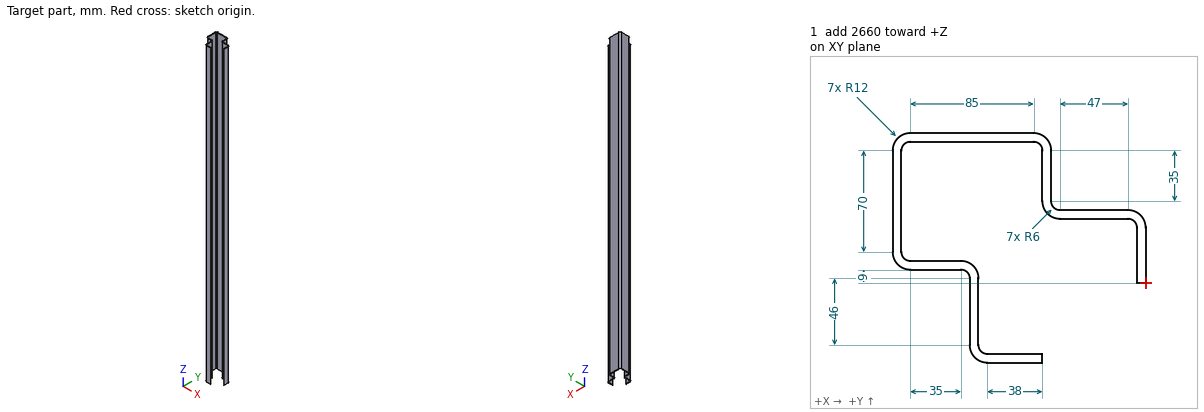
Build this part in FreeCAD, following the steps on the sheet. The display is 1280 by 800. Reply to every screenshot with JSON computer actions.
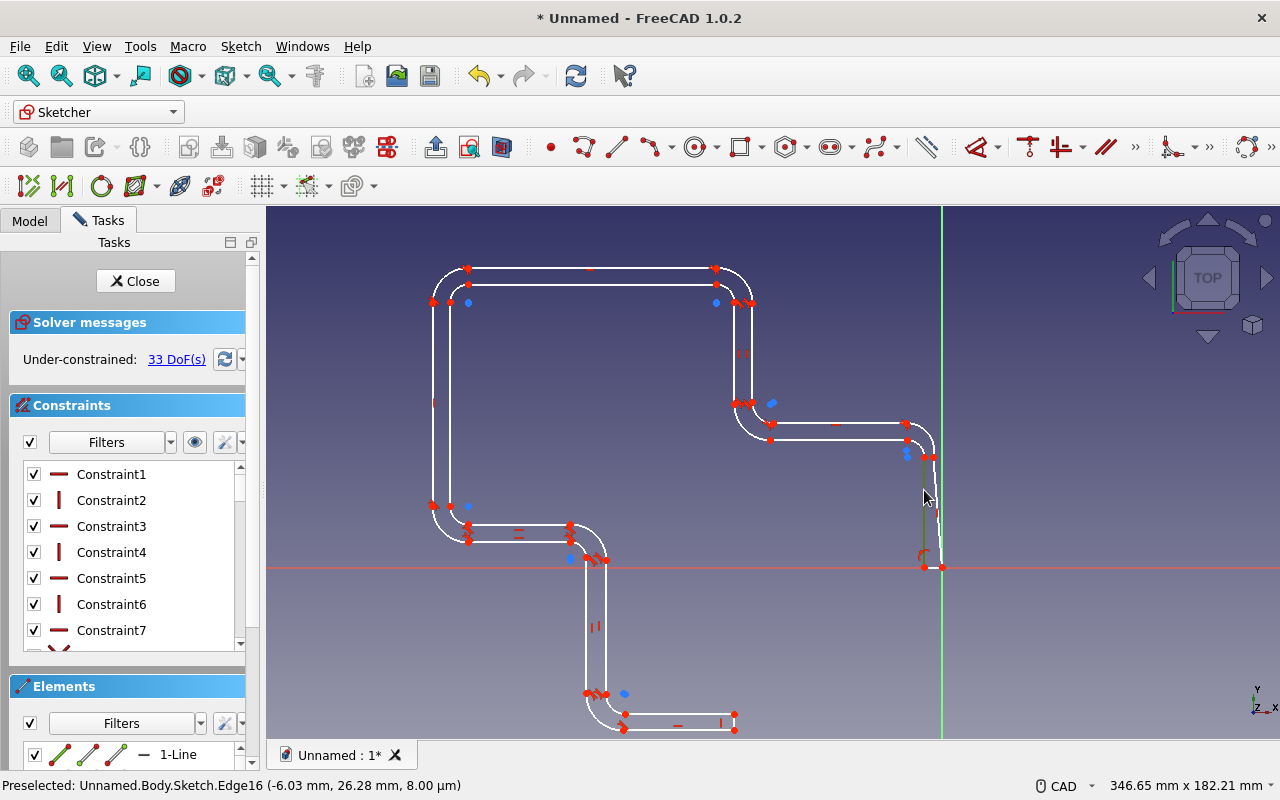
{"action": "left_click", "coordinate": [919, 445]}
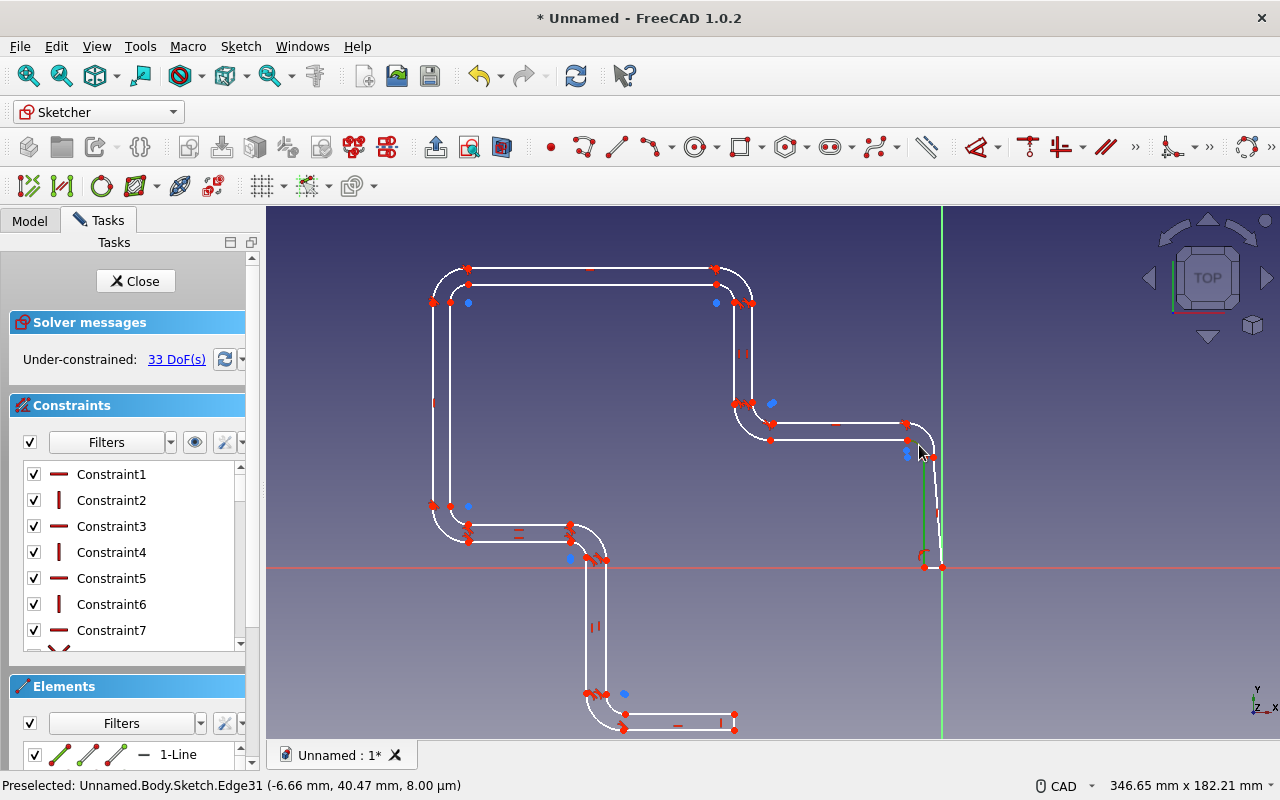
{"action": "key", "text": "t"}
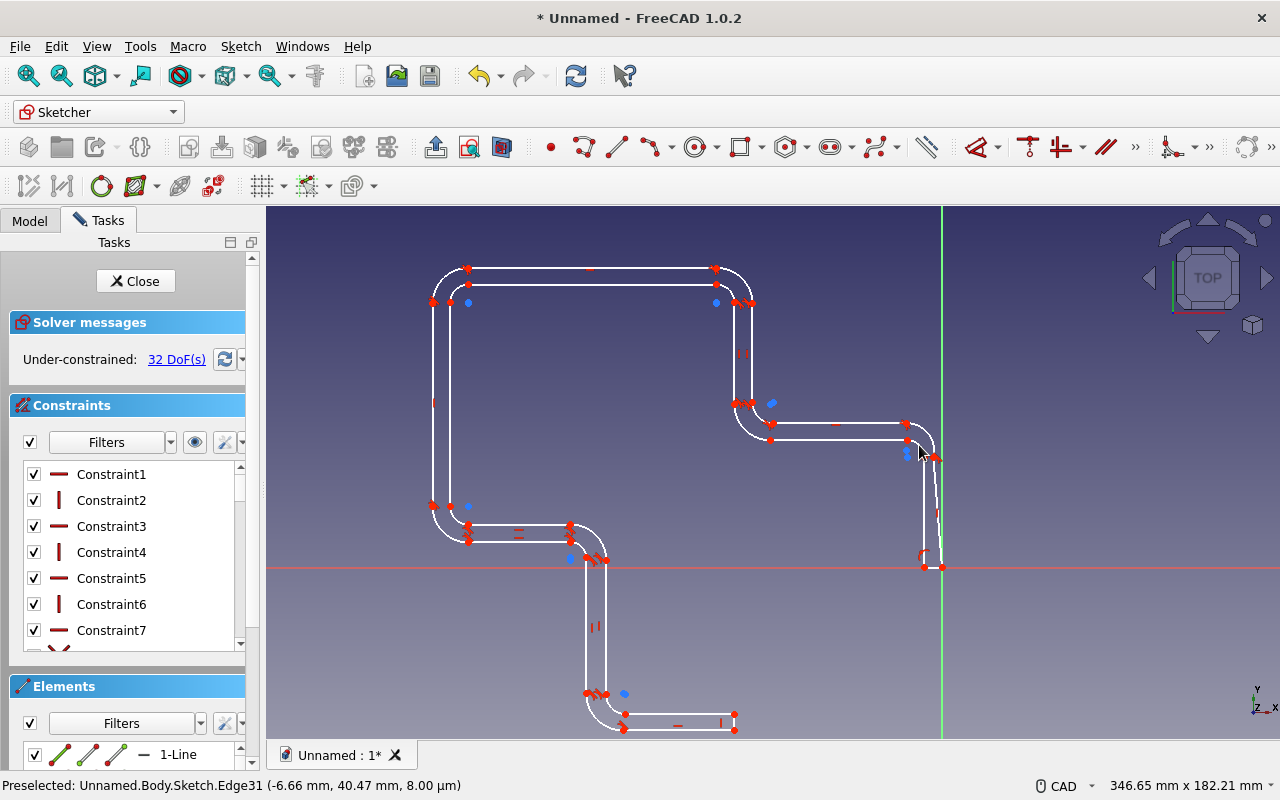
{"action": "left_click", "coordinate": [939, 535]}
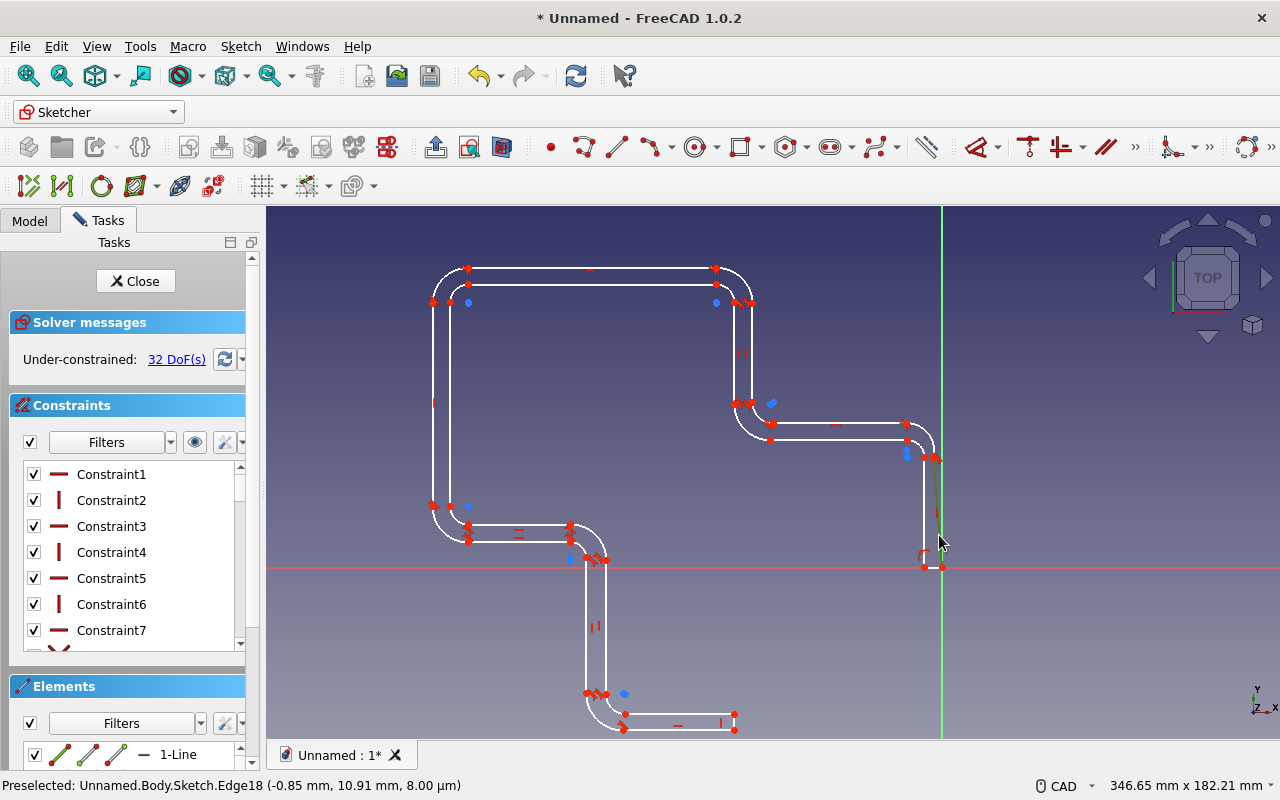
{"action": "scroll", "coordinate": [933, 442], "scroll_direction": "up", "scroll_amount": 3}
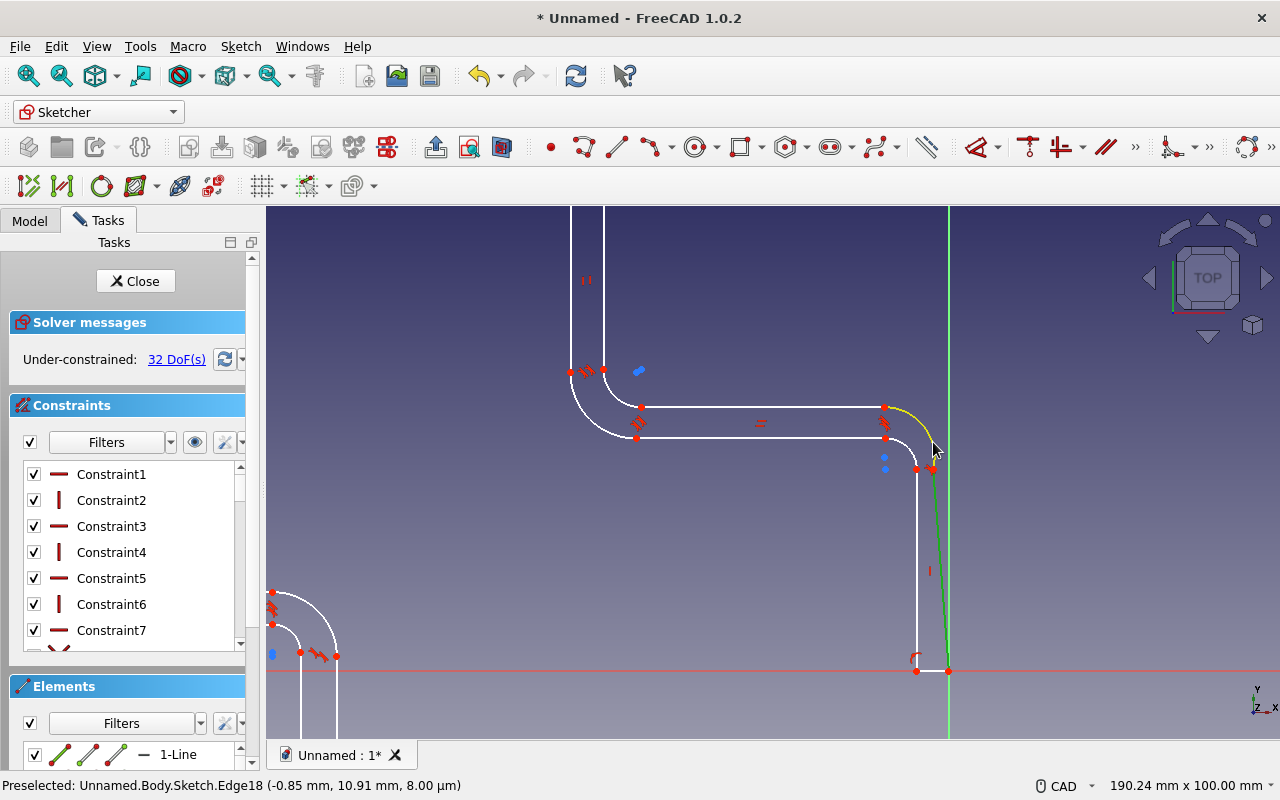
{"action": "left_click", "coordinate": [932, 442]}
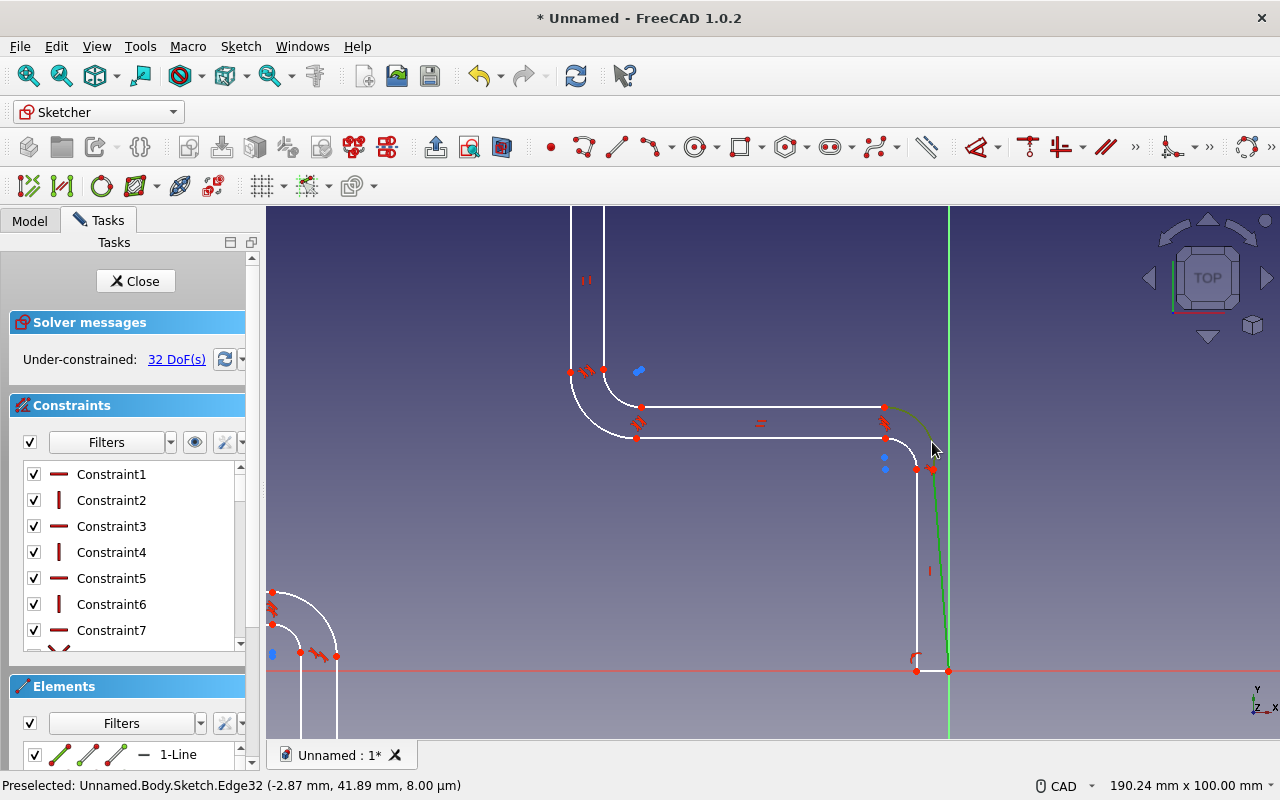
{"action": "key", "text": "t"}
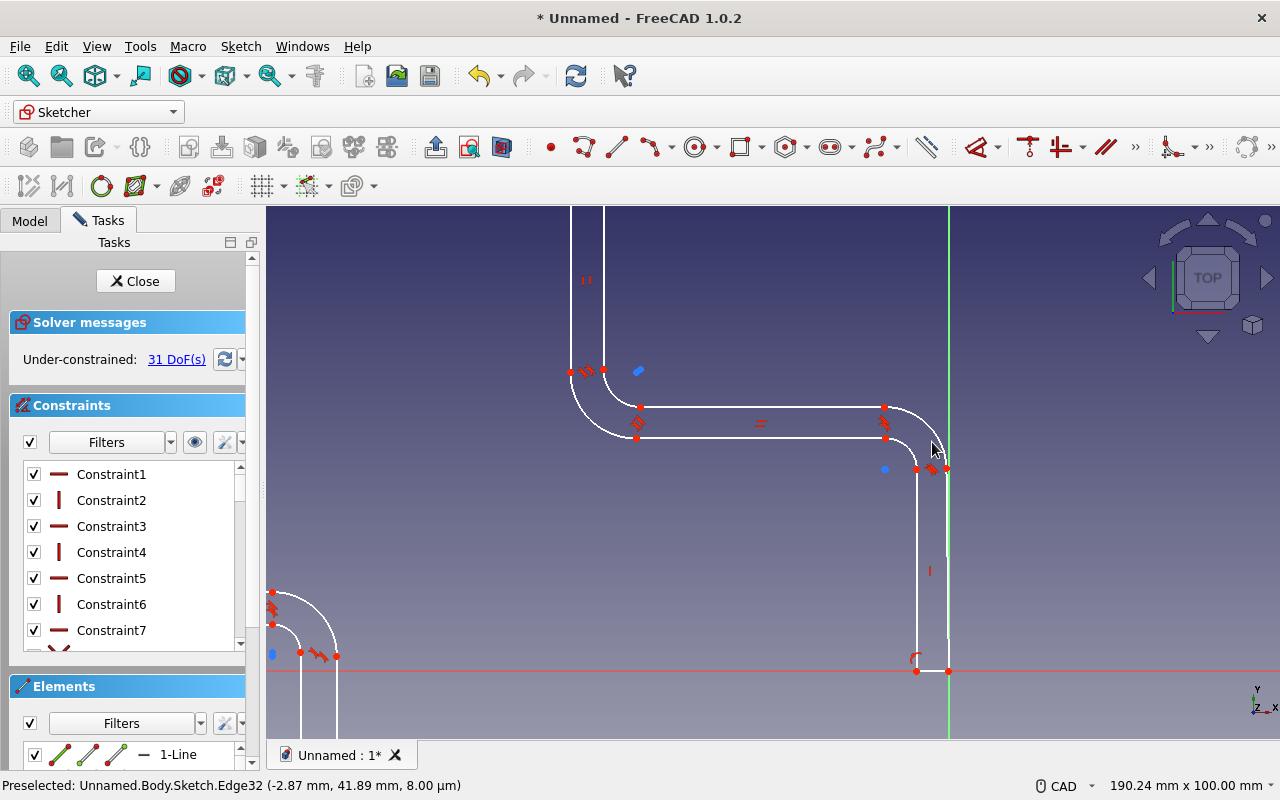
{"action": "left_click", "coordinate": [948, 610]}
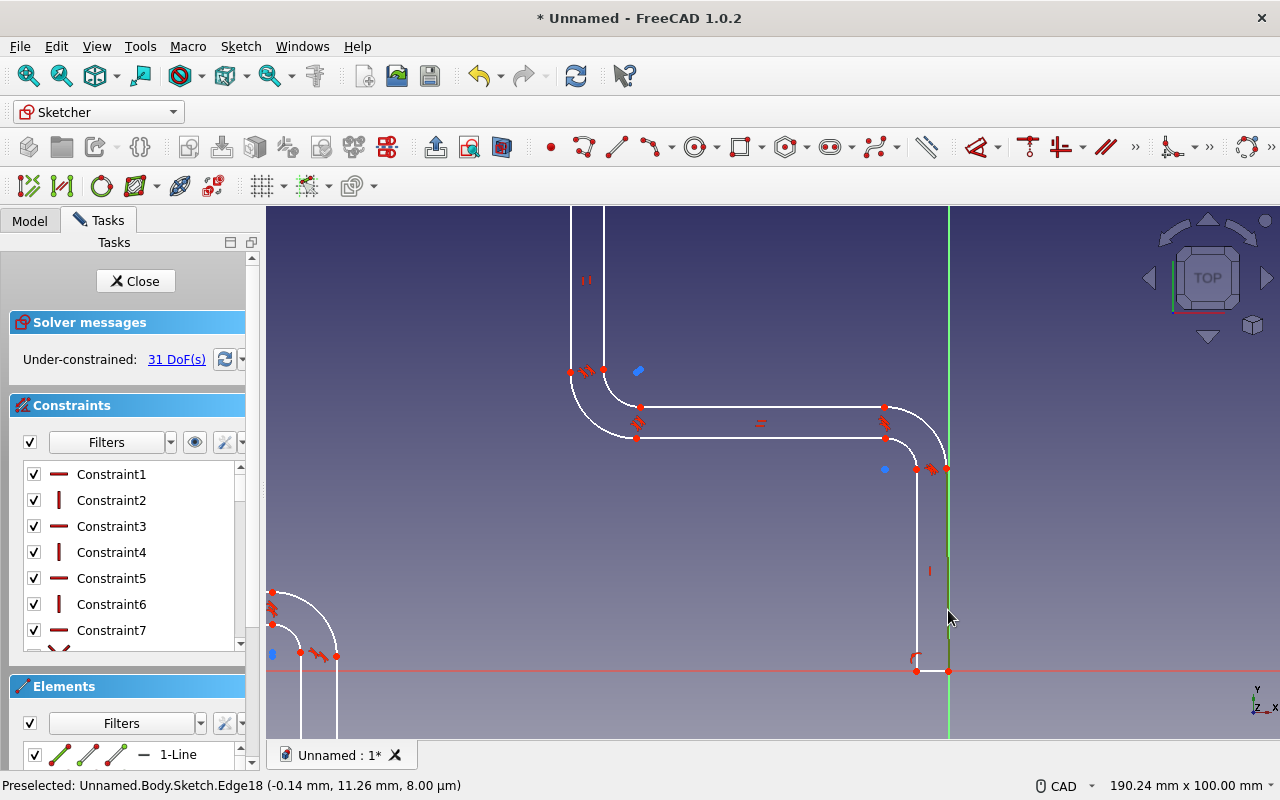
{"action": "key", "text": "v"}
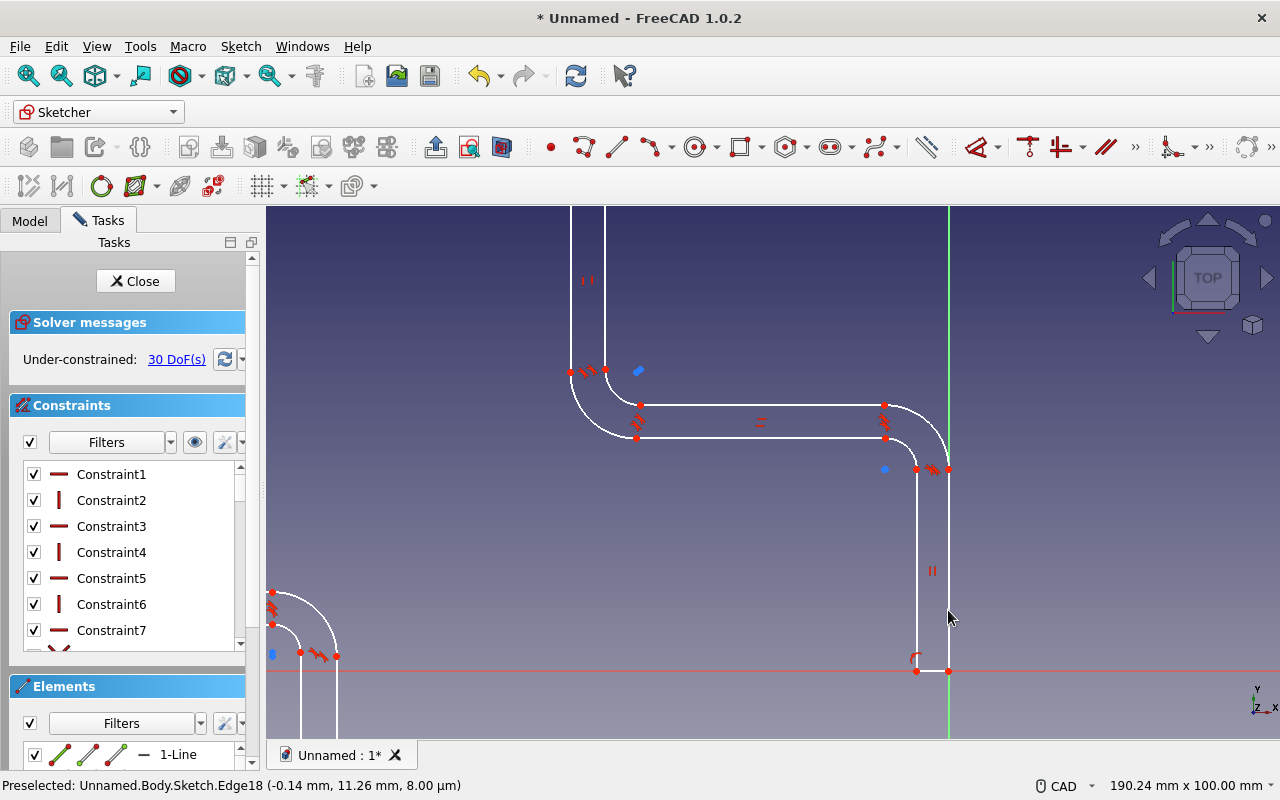
{"action": "scroll", "coordinate": [832, 431], "scroll_direction": "down", "scroll_amount": 5}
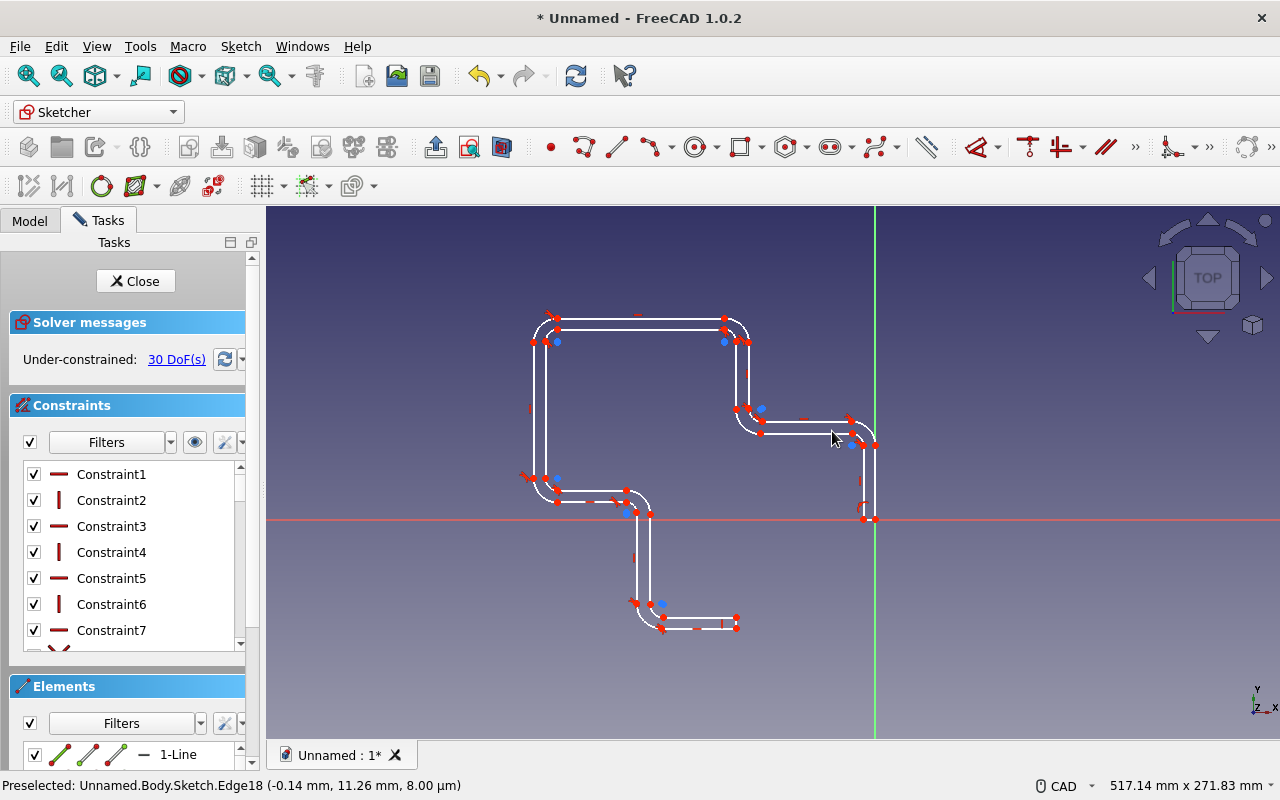
{"action": "left_click", "coordinate": [640, 615]}